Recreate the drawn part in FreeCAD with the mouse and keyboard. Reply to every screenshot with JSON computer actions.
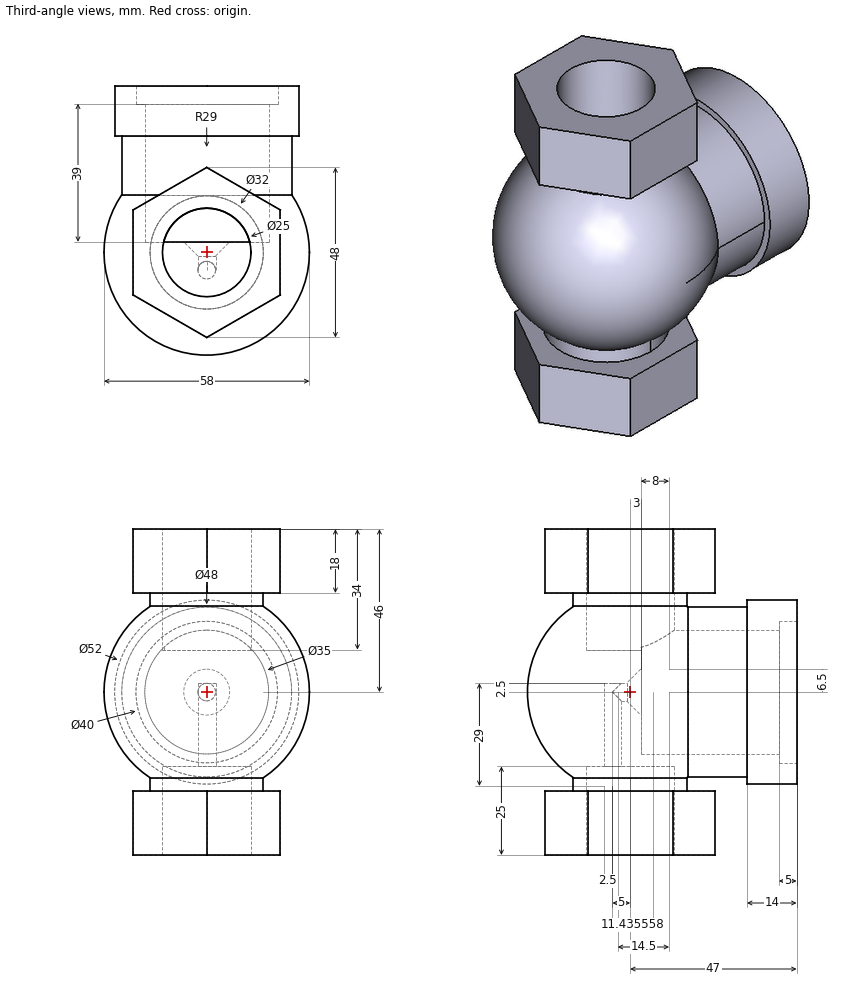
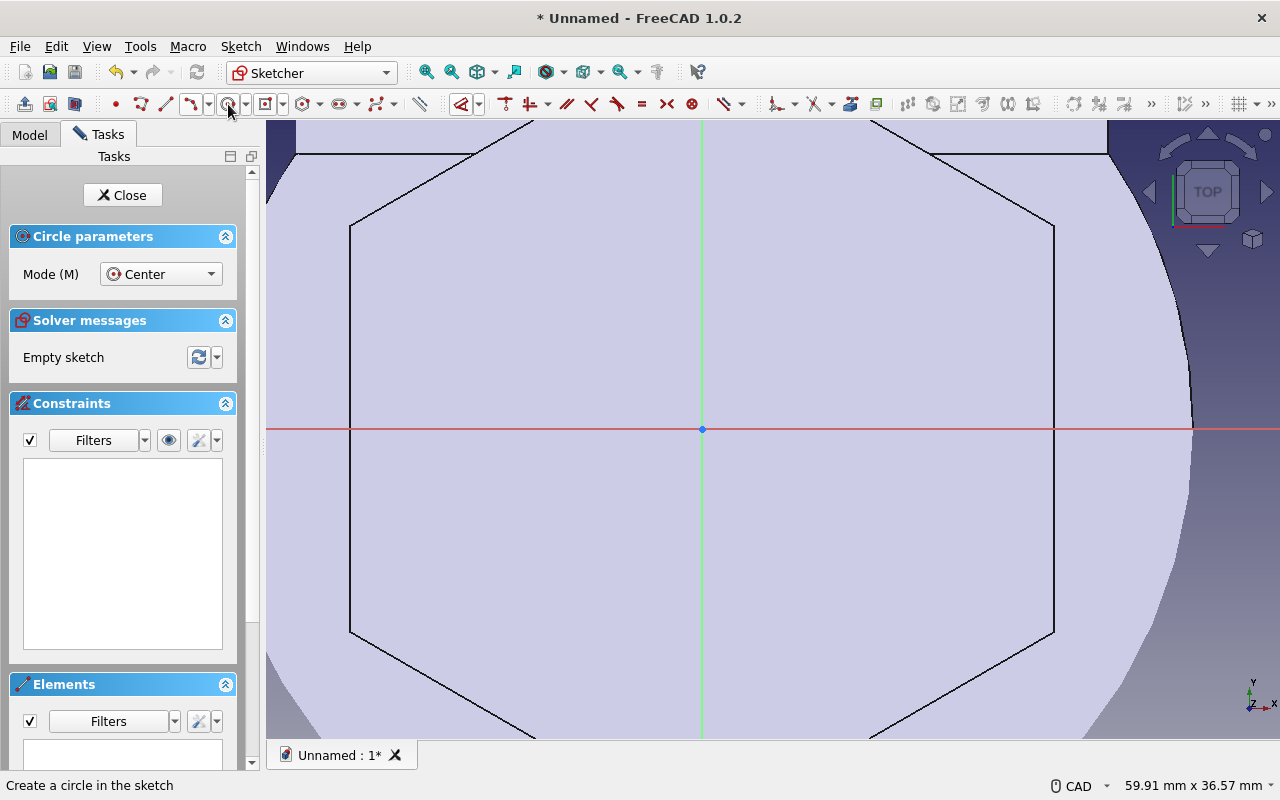
{"action": "left_click", "coordinate": [702, 429]}
{"action": "left_click", "coordinate": [852, 279]}
{"action": "key", "text": "Escape"}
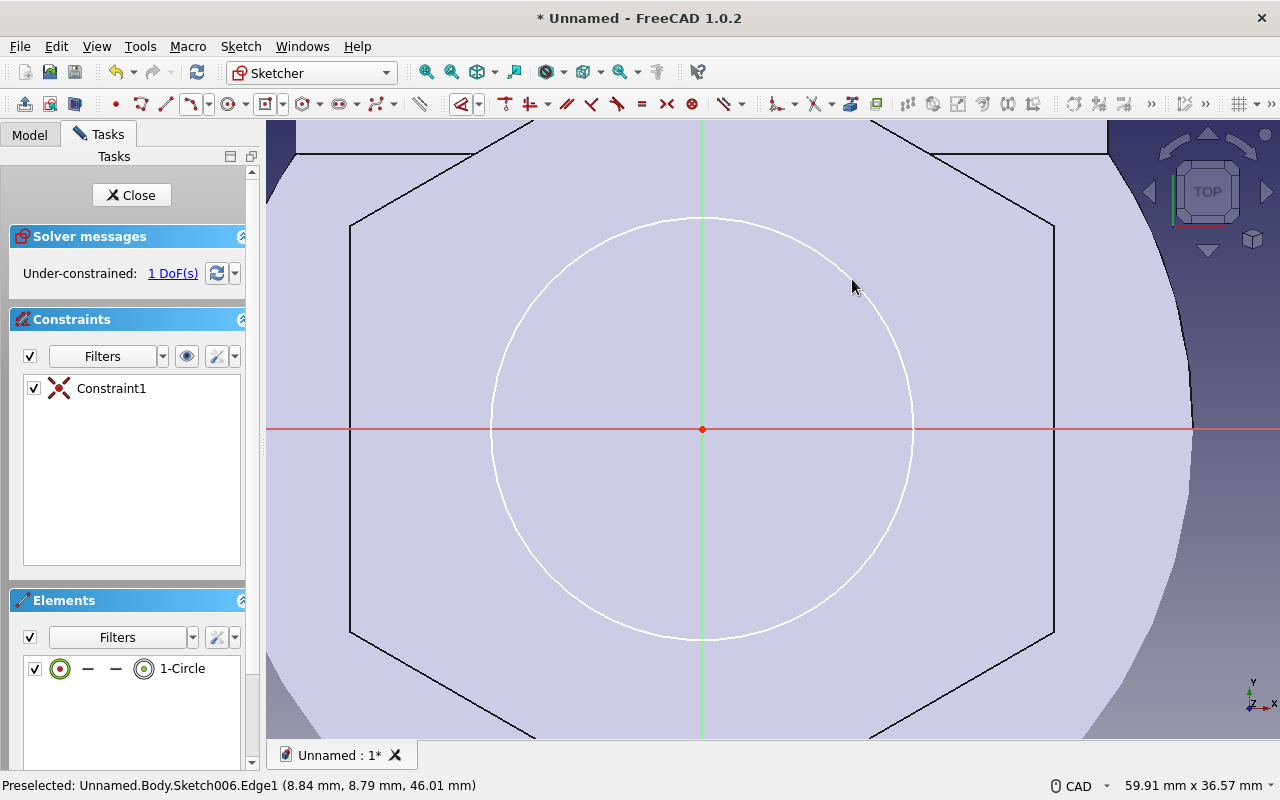
{"action": "left_click", "coordinate": [851, 279]}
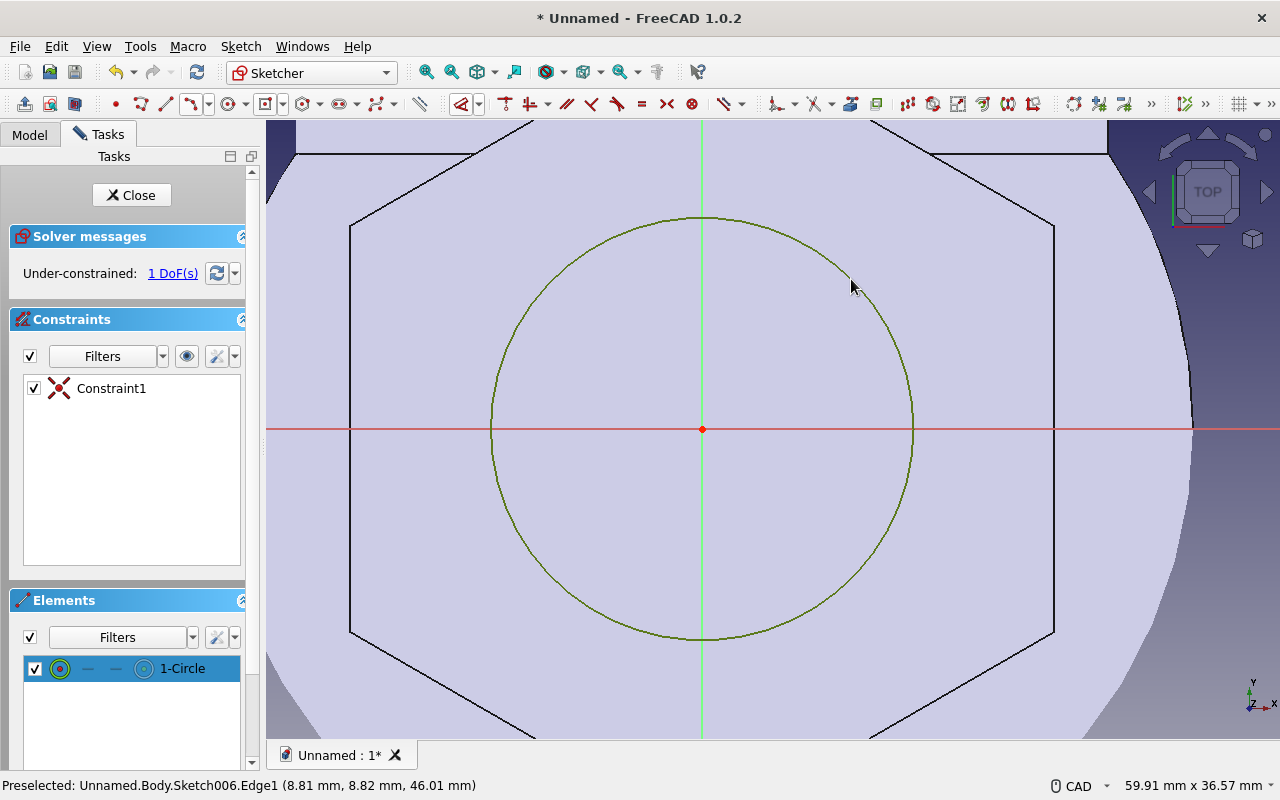
{"action": "left_click", "coordinate": [478, 104]}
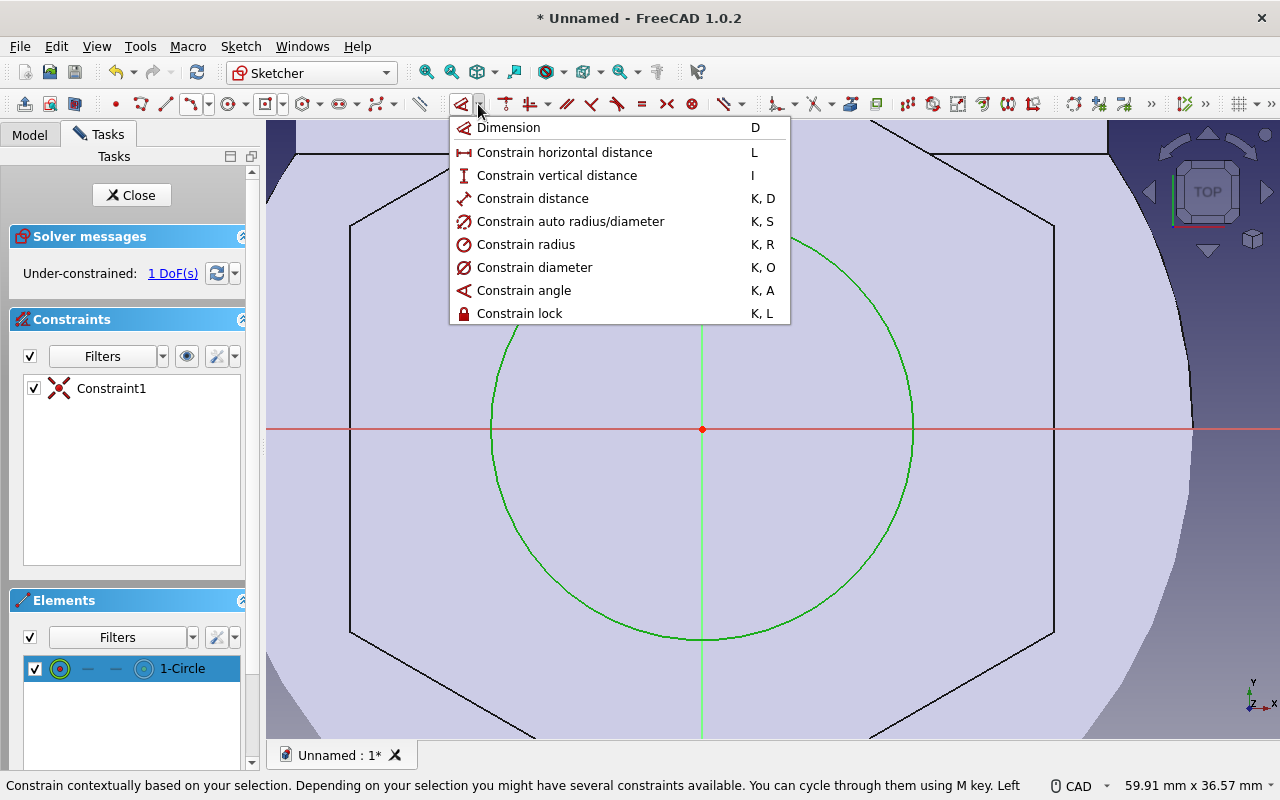
{"action": "left_click", "coordinate": [620, 268]}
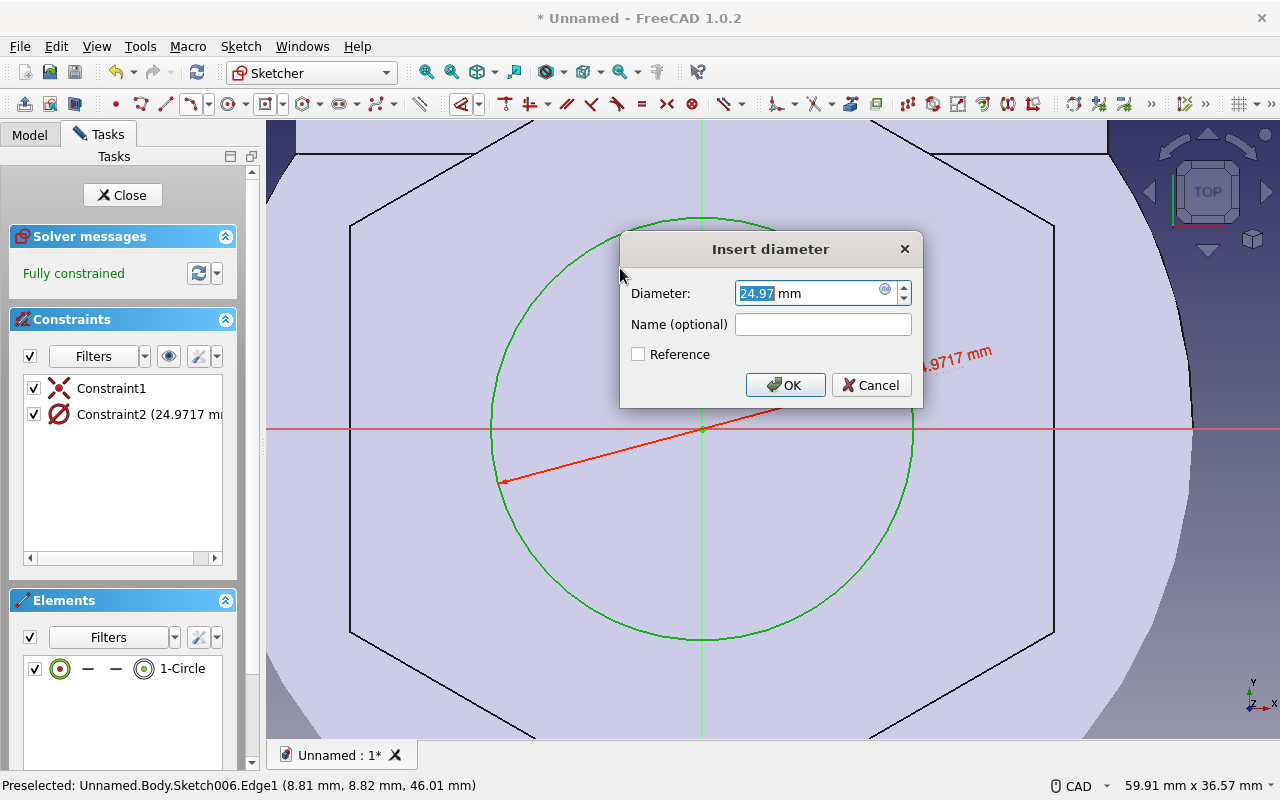
{"action": "type", "text": "25"}
{"action": "key", "text": "Return"}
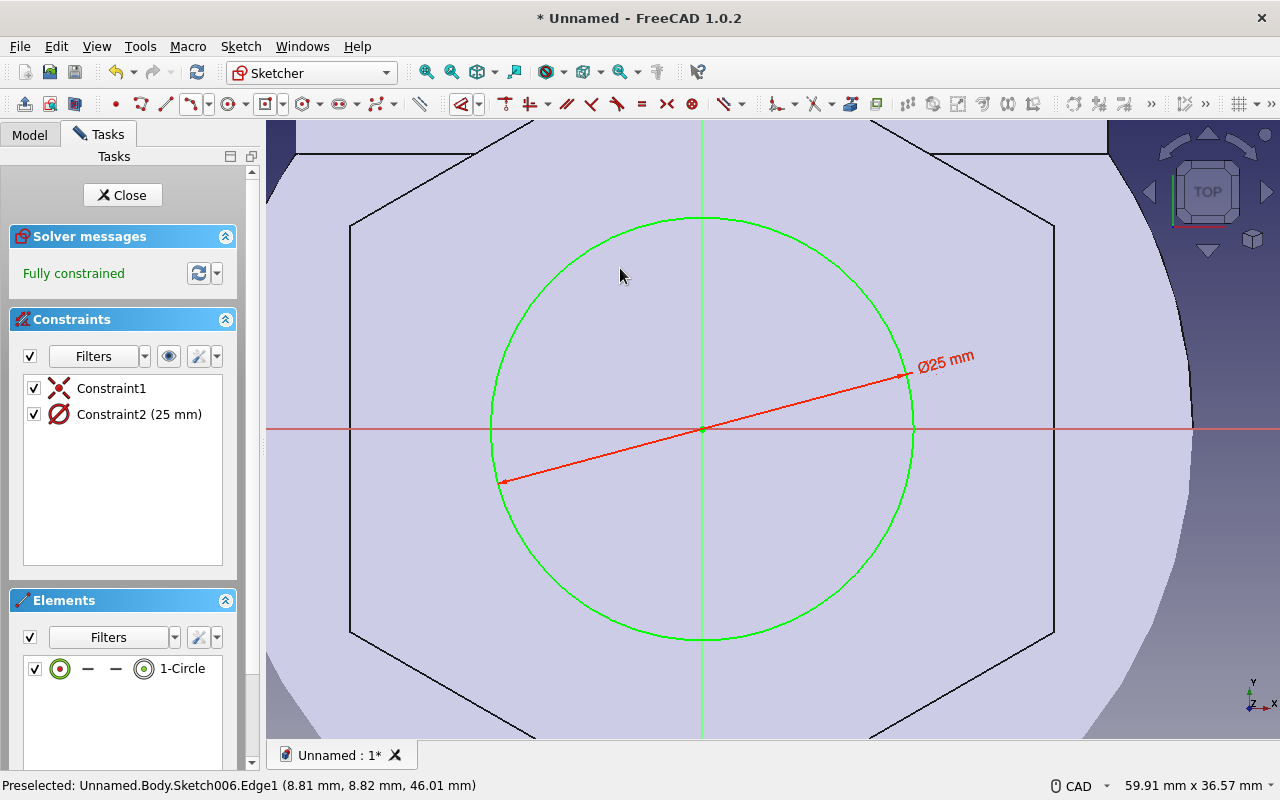
{"action": "left_click", "coordinate": [123, 195]}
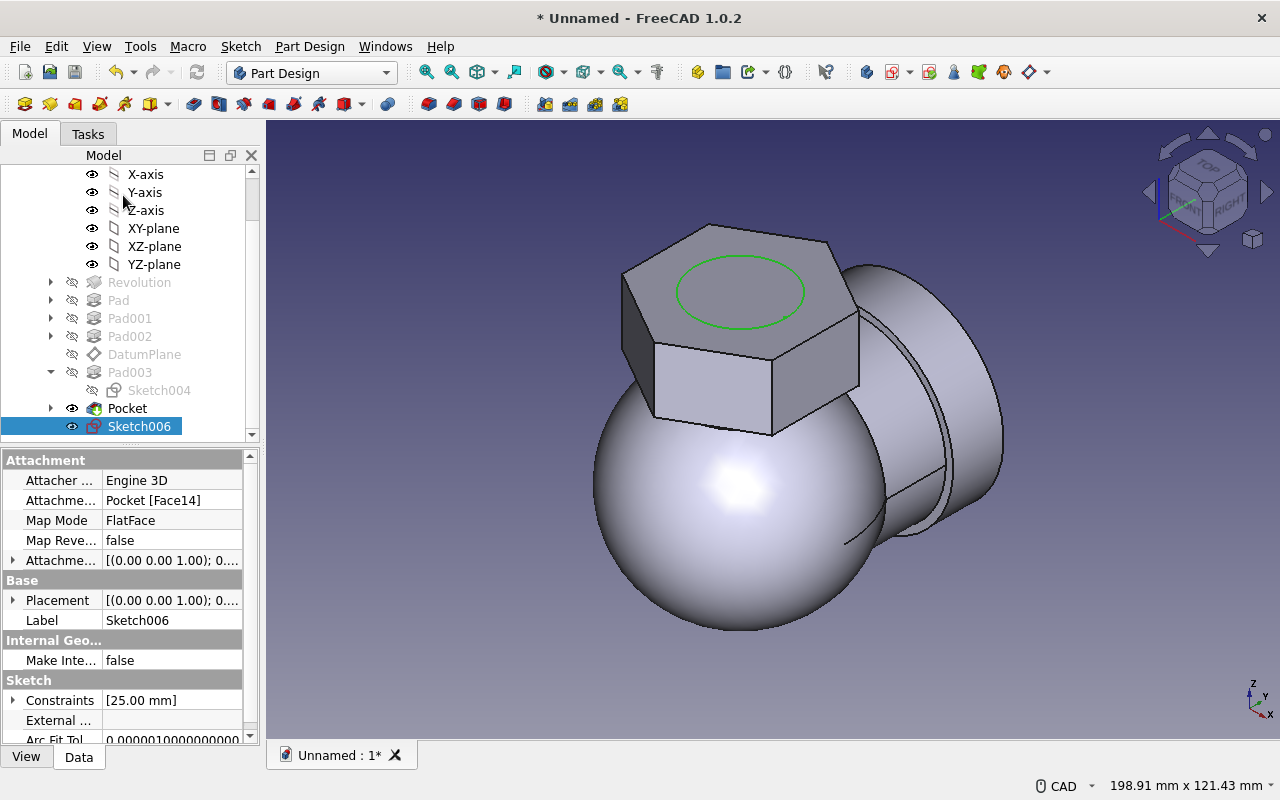
{"action": "left_click", "coordinate": [194, 104]}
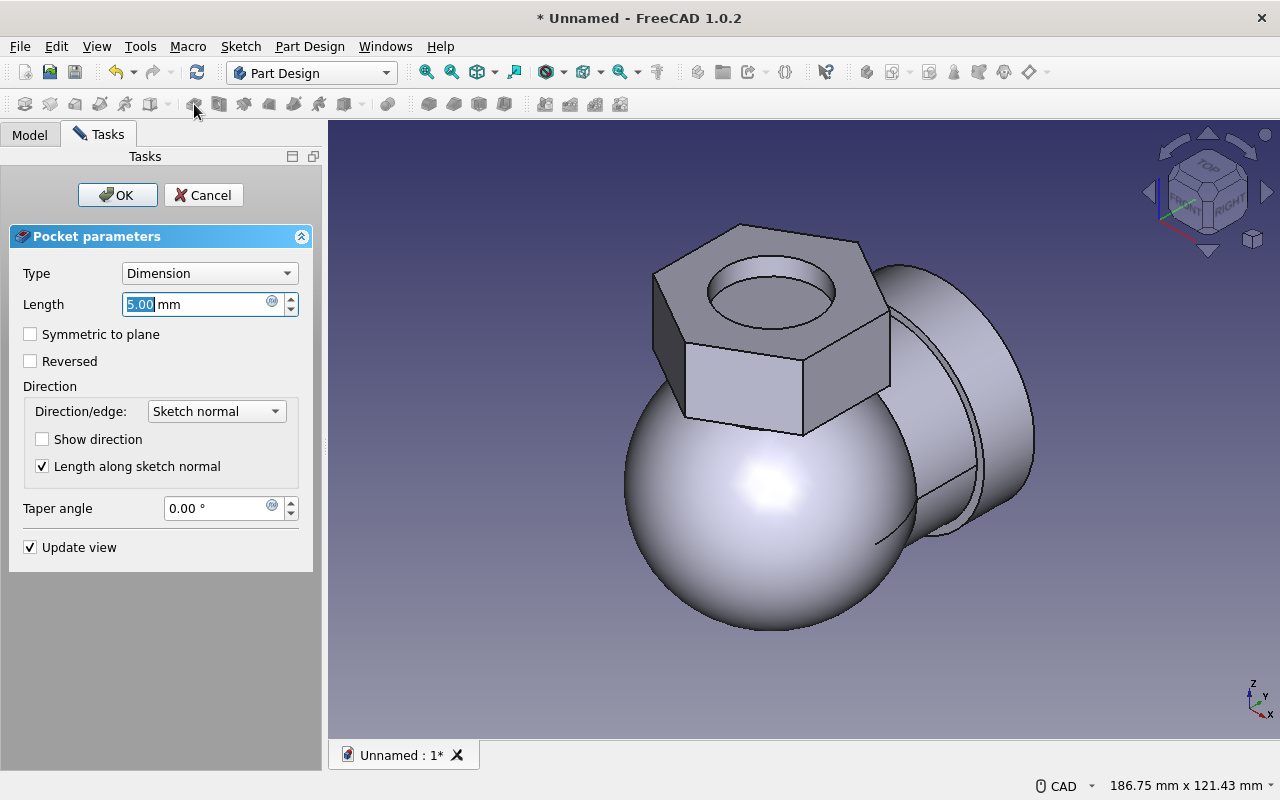
{"action": "type", "text": "34"}
{"action": "key", "text": "Tab"}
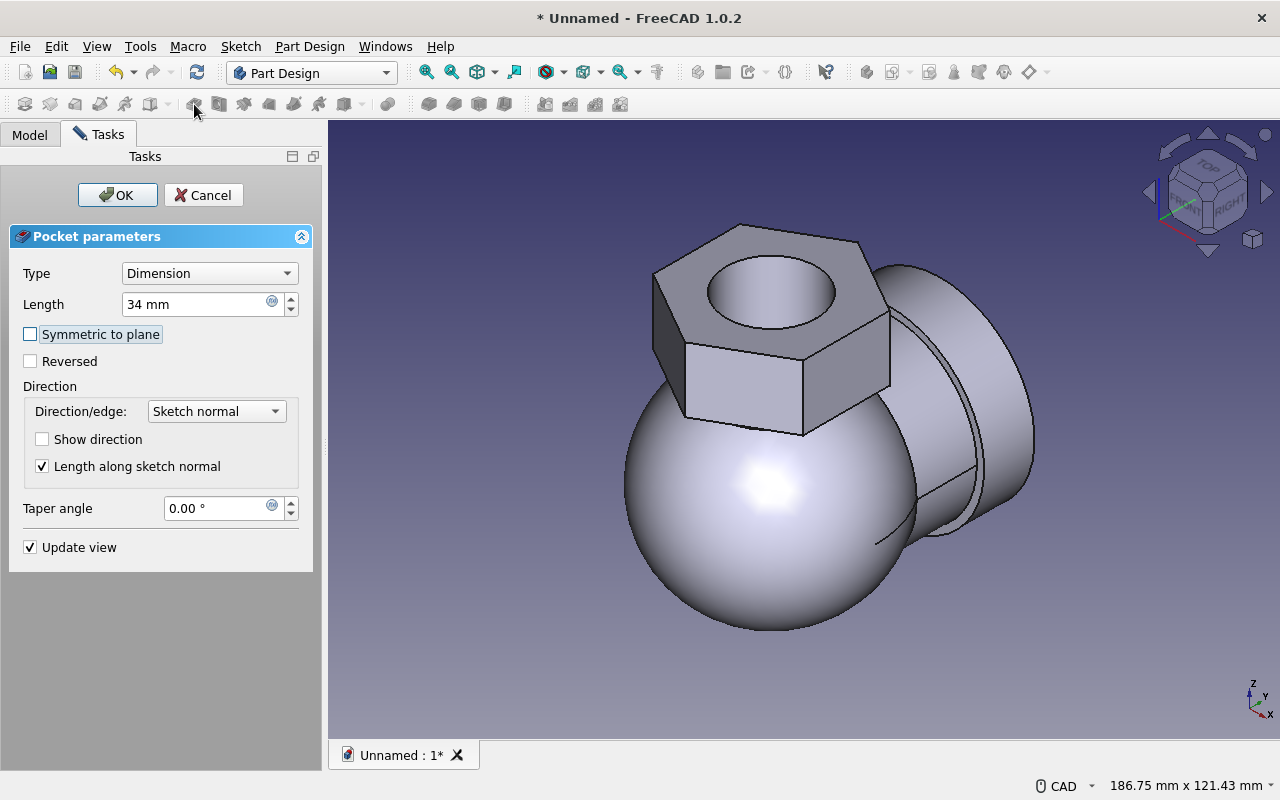
{"action": "left_click", "coordinate": [118, 195]}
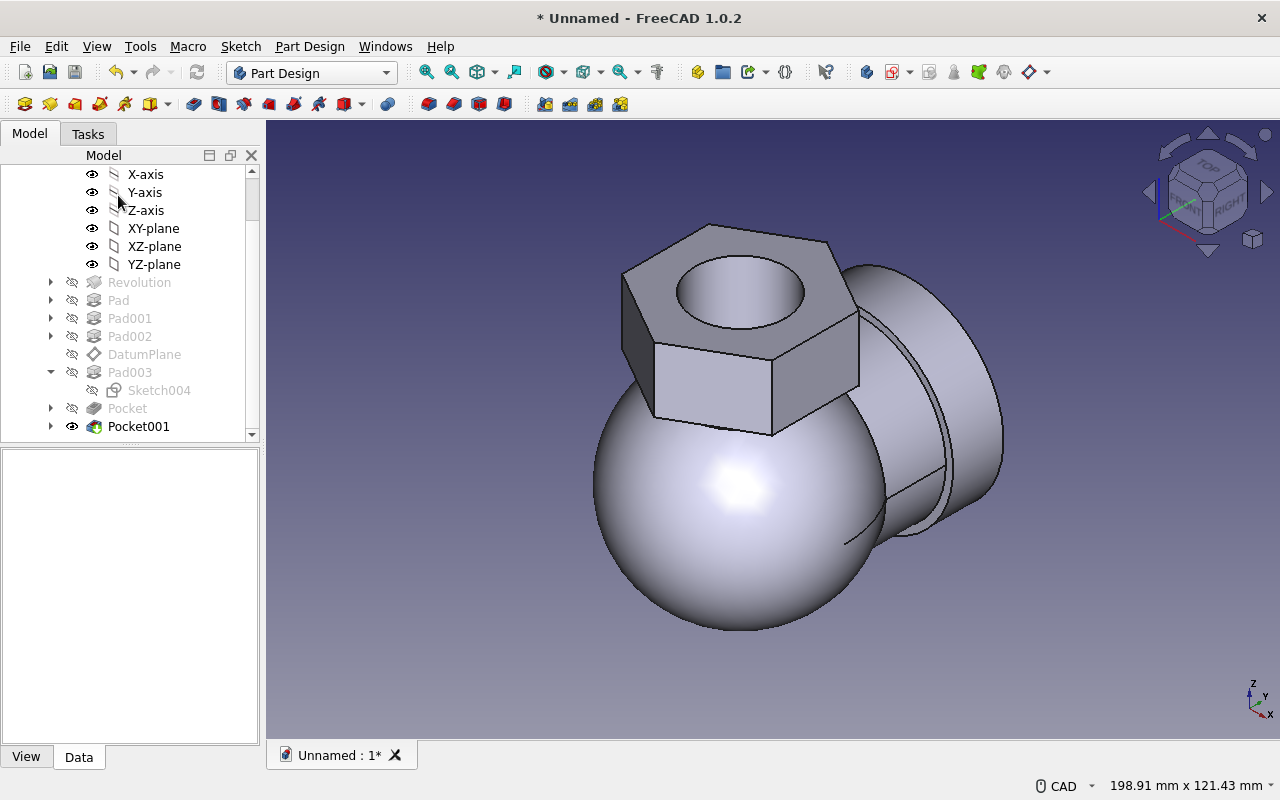
{"action": "left_click", "coordinate": [117, 336]}